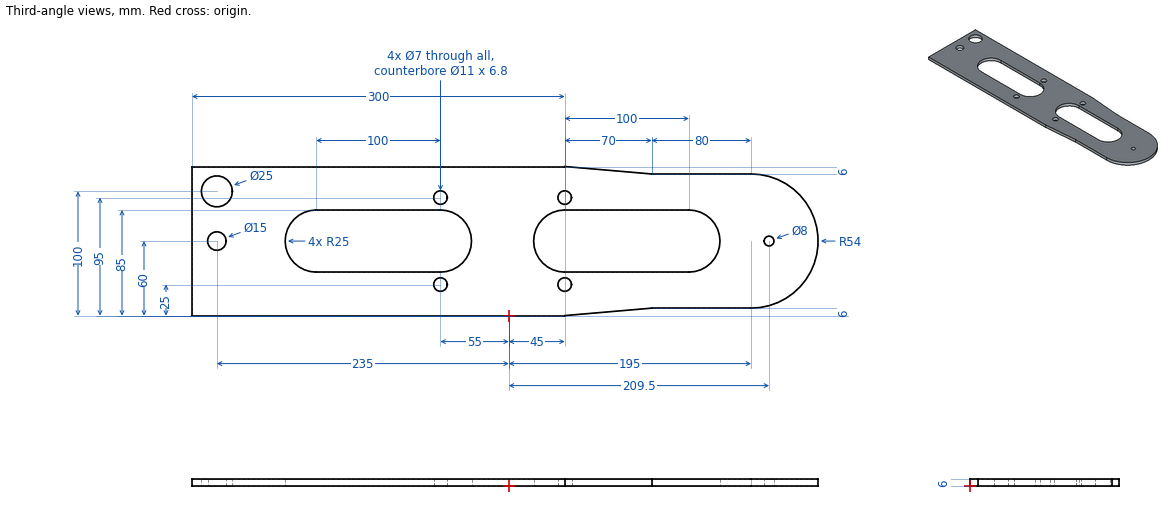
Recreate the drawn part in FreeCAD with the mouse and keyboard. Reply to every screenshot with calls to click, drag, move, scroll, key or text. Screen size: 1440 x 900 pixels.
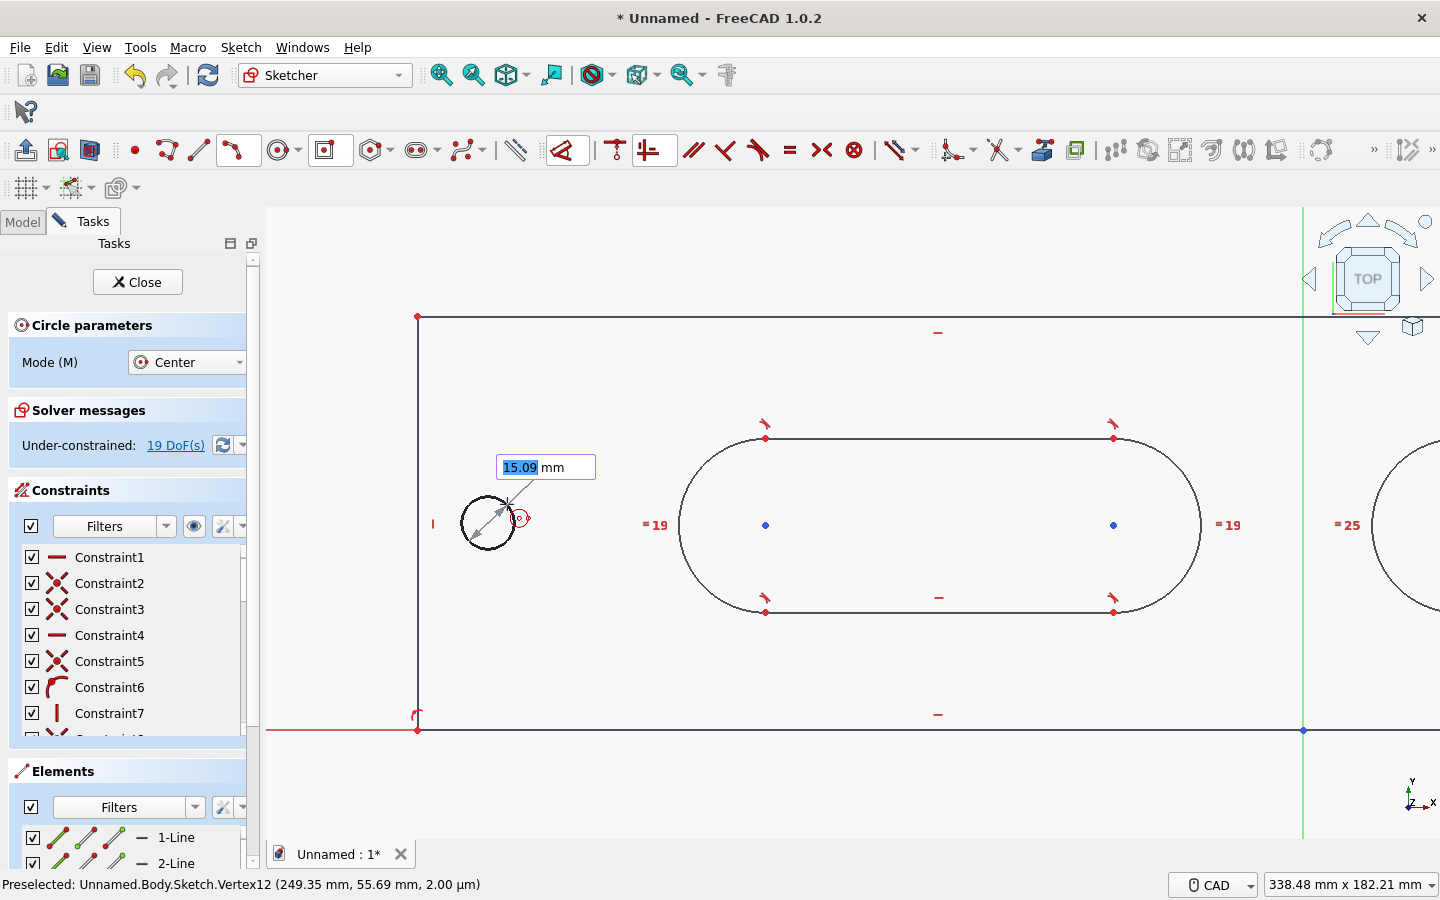
text(15)
key(Return)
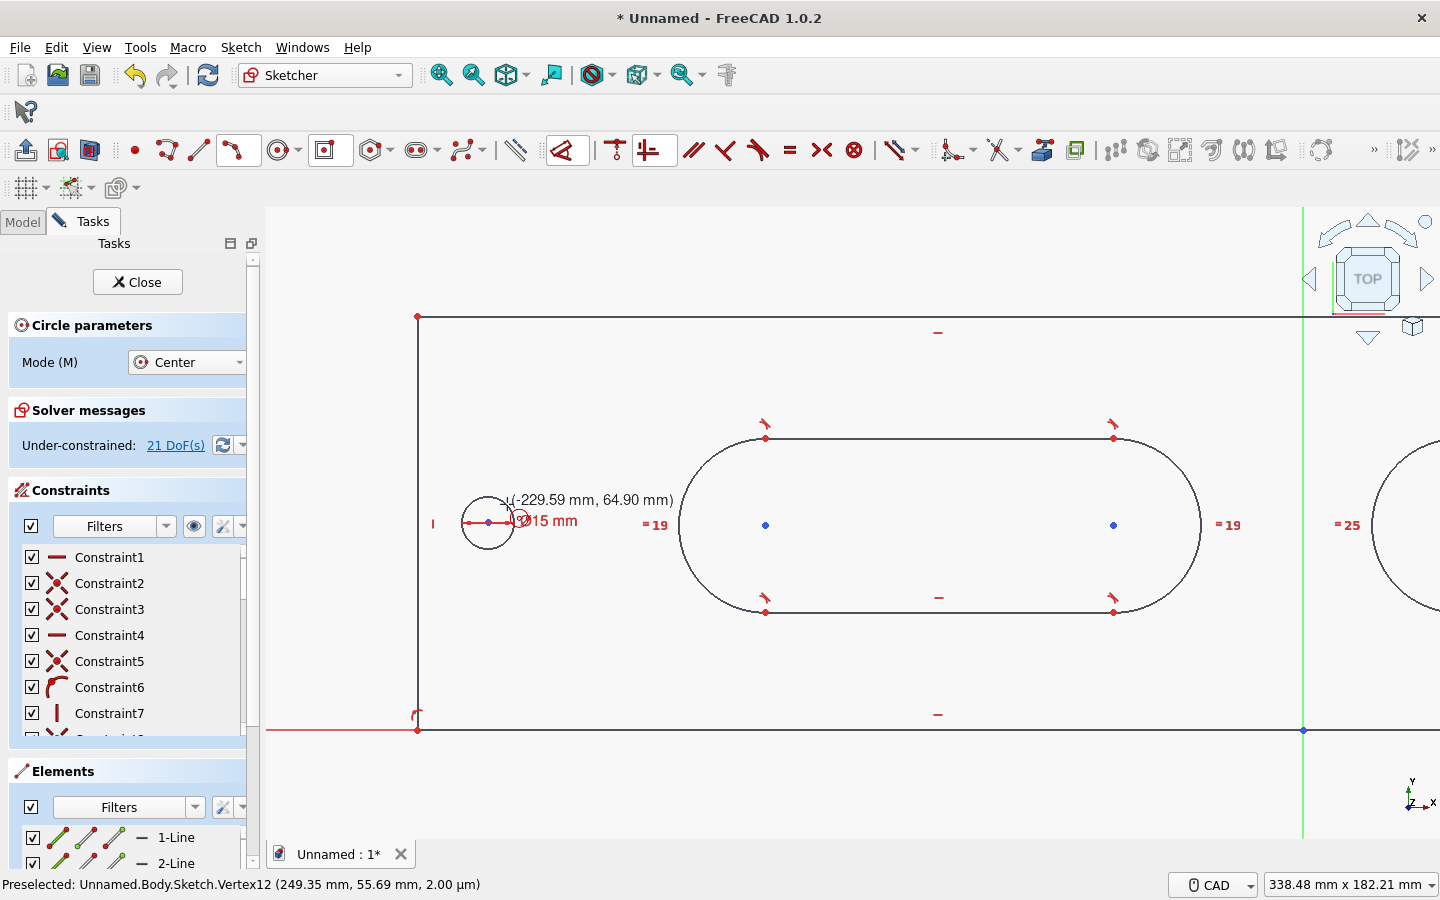
click(488, 383)
move(519, 353)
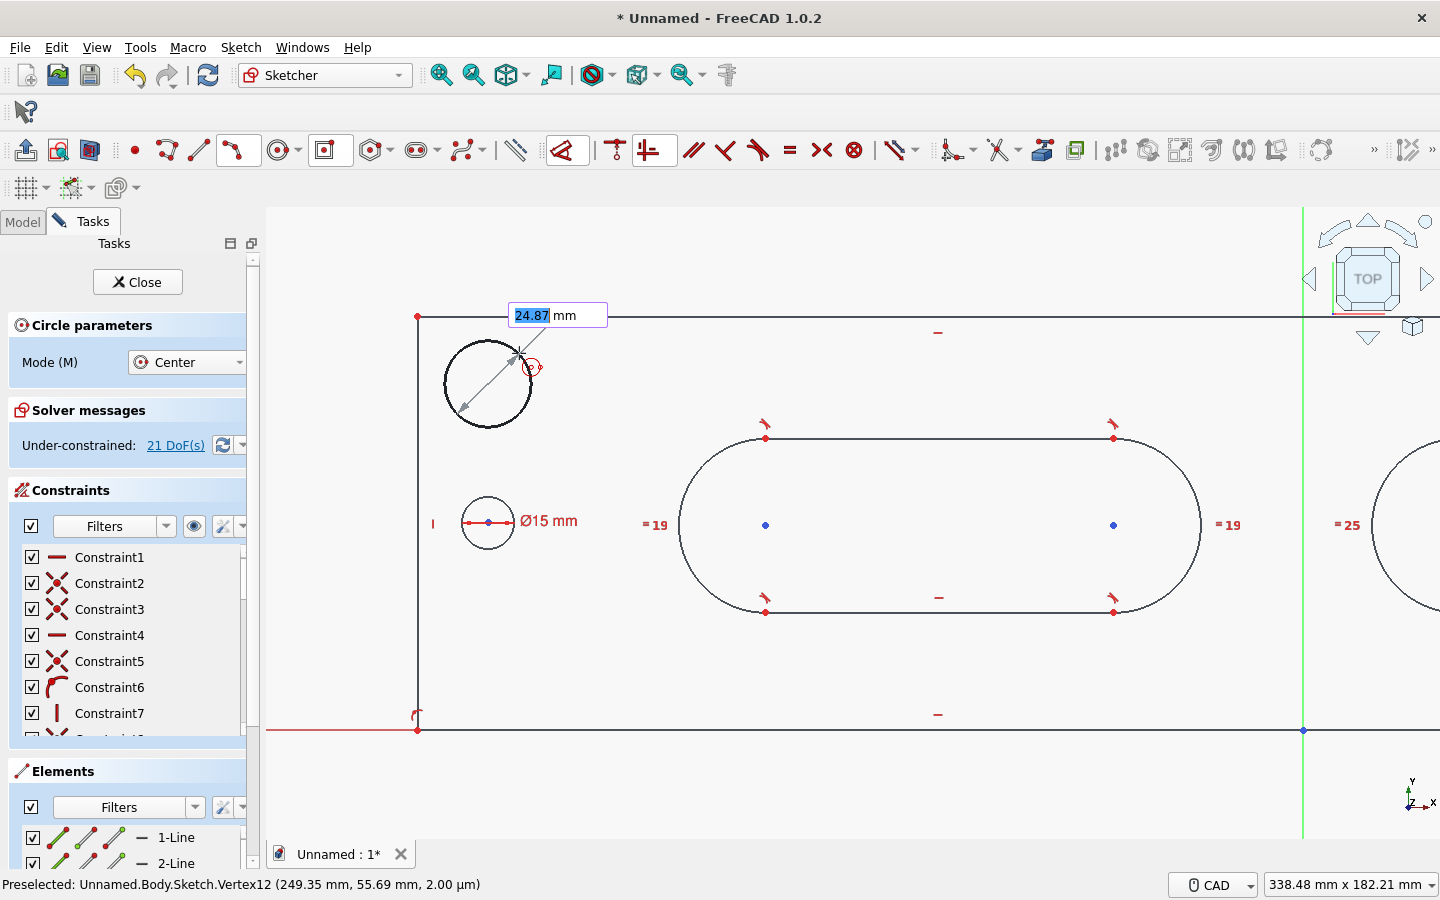
text(25)
key(Return)
key(Escape)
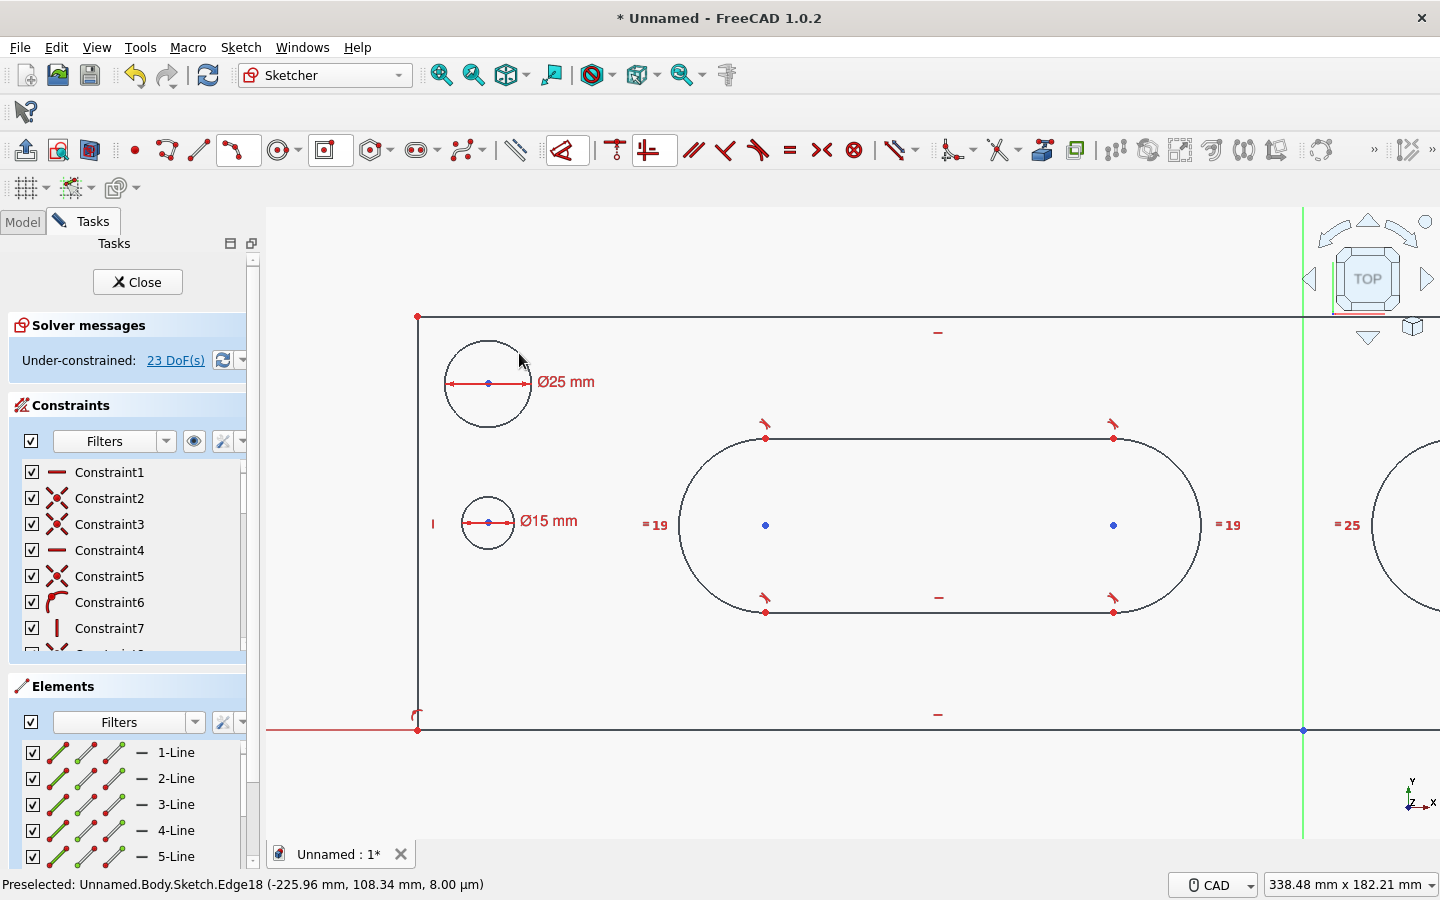
click(696, 475)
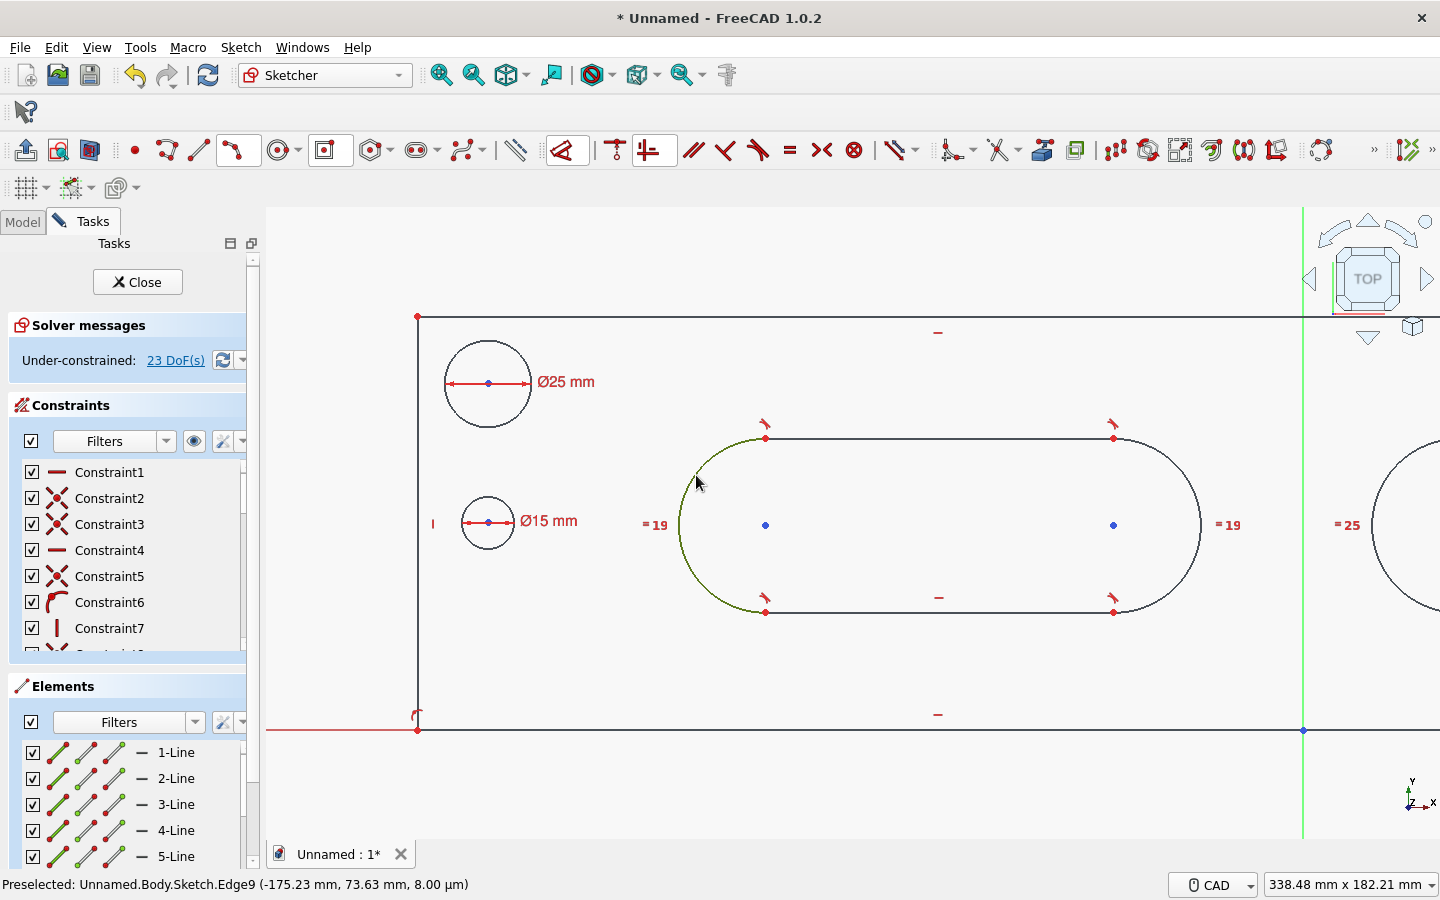
scroll(489, 524, down, 5)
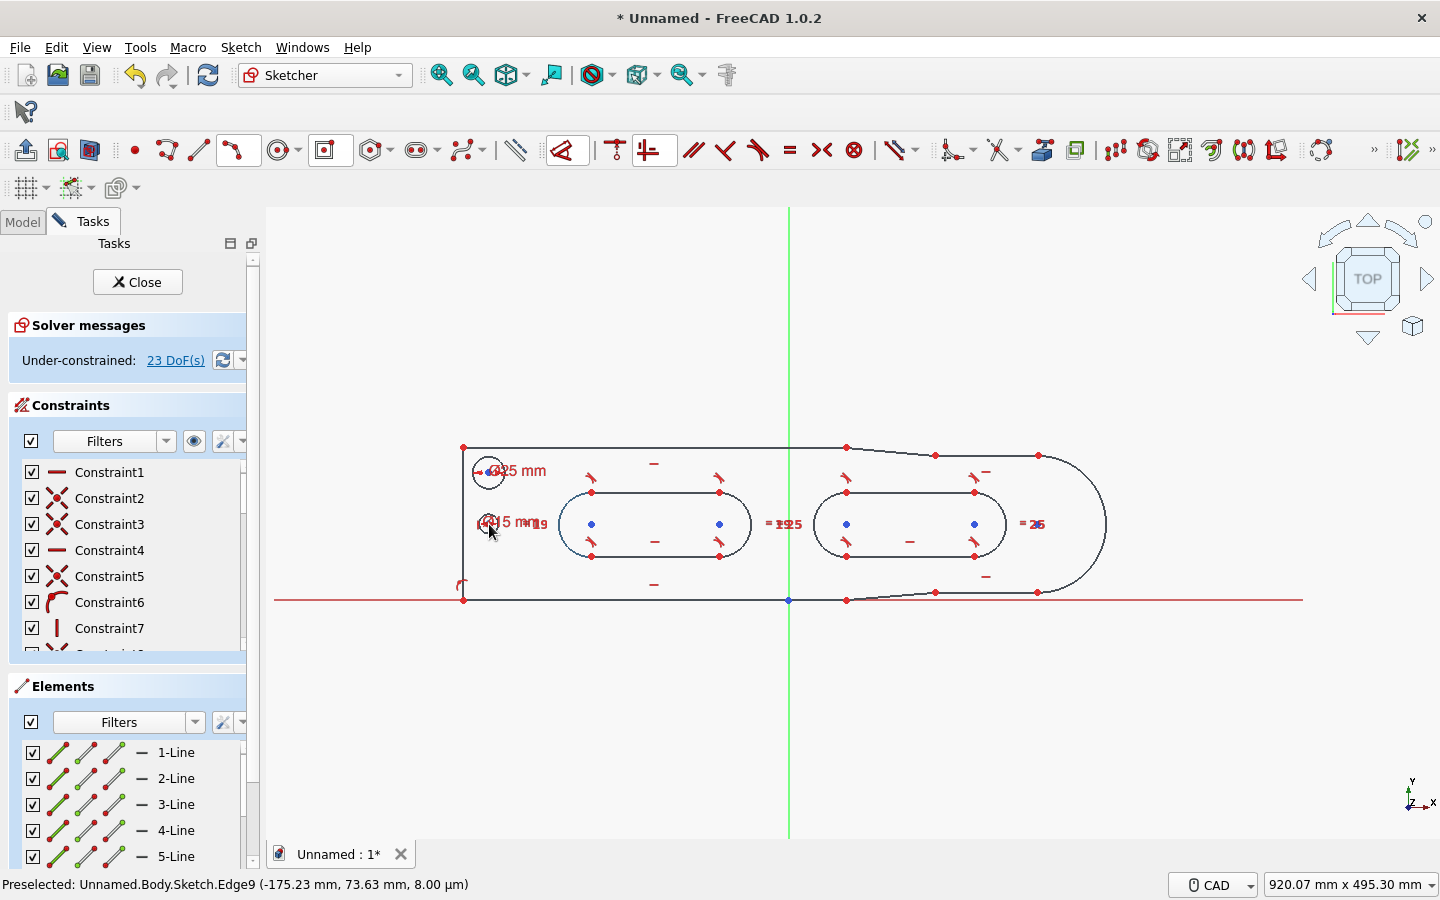
click(820, 506)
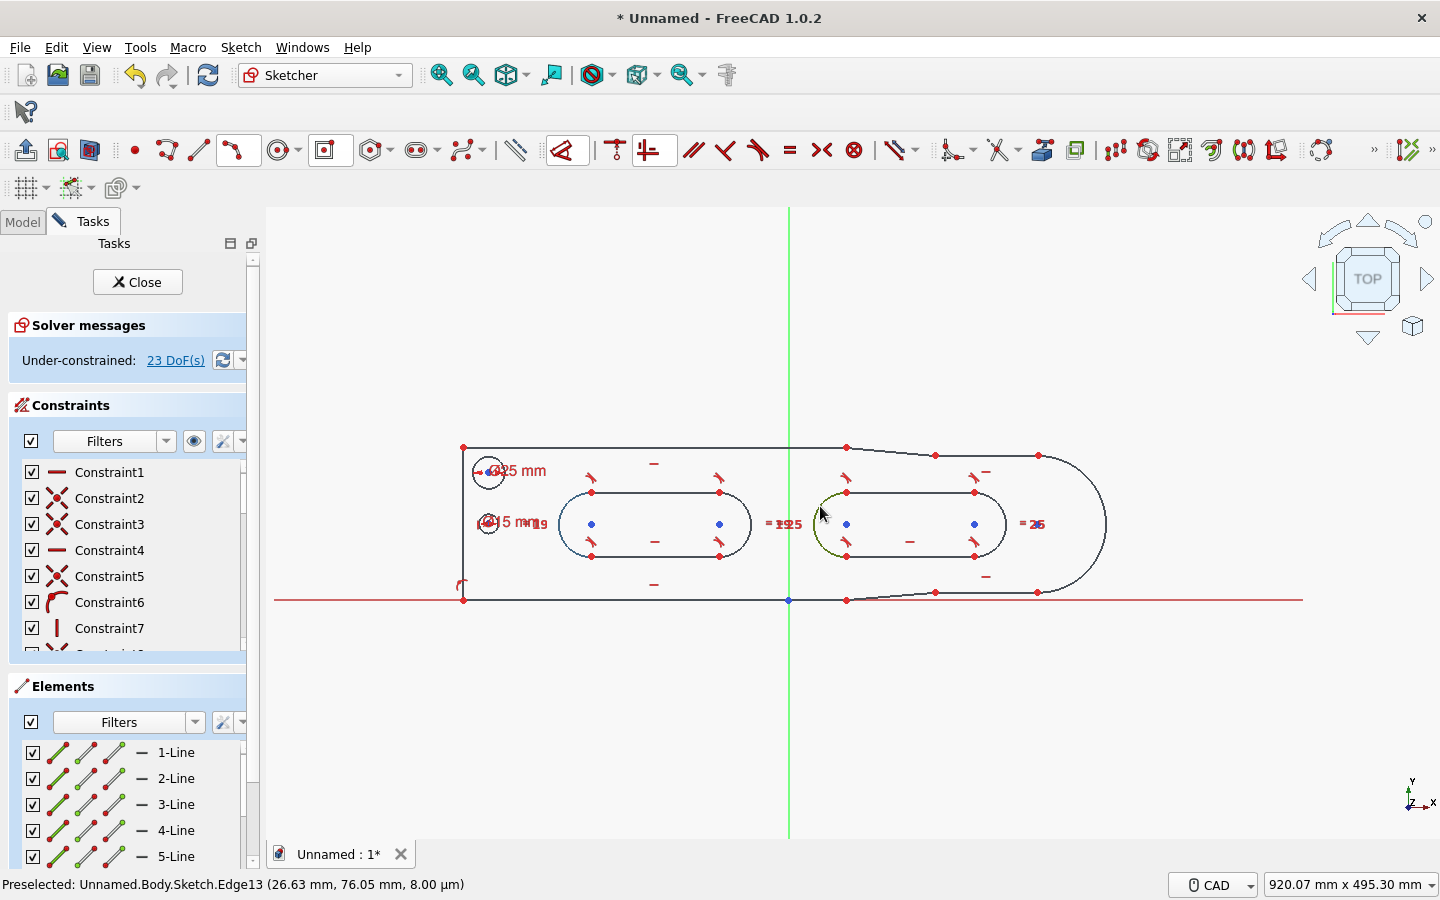
key(e)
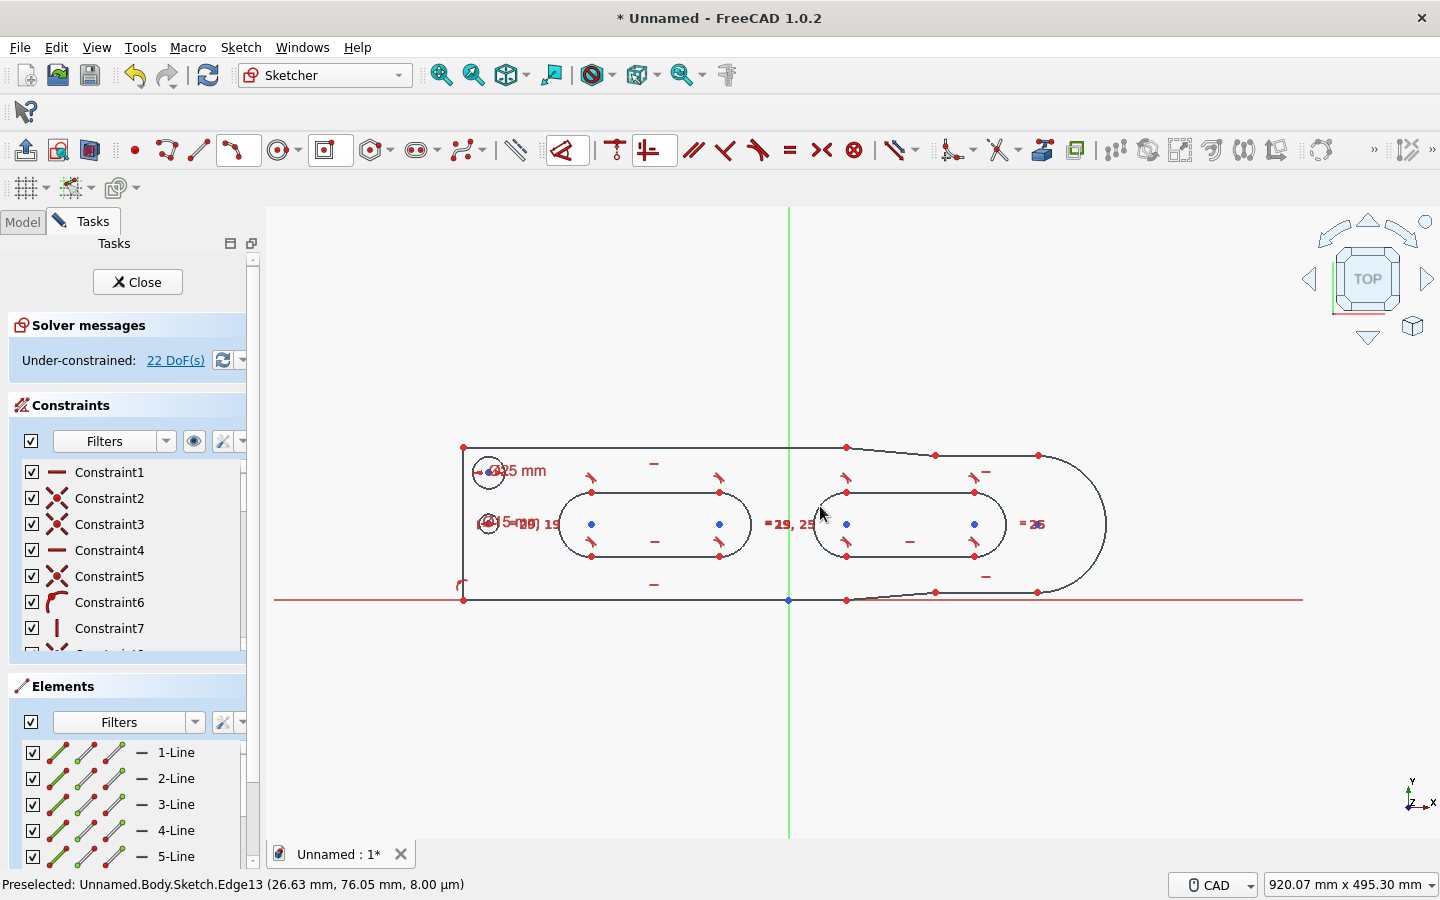
click(489, 524)